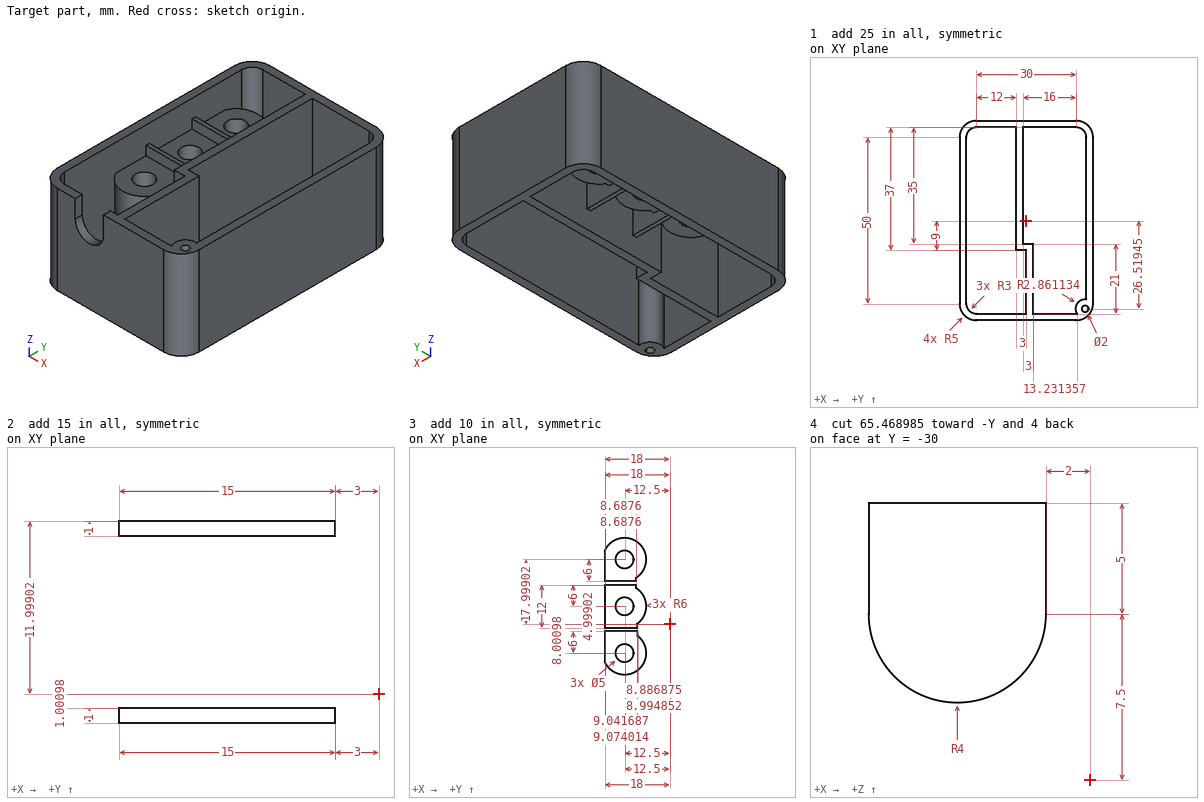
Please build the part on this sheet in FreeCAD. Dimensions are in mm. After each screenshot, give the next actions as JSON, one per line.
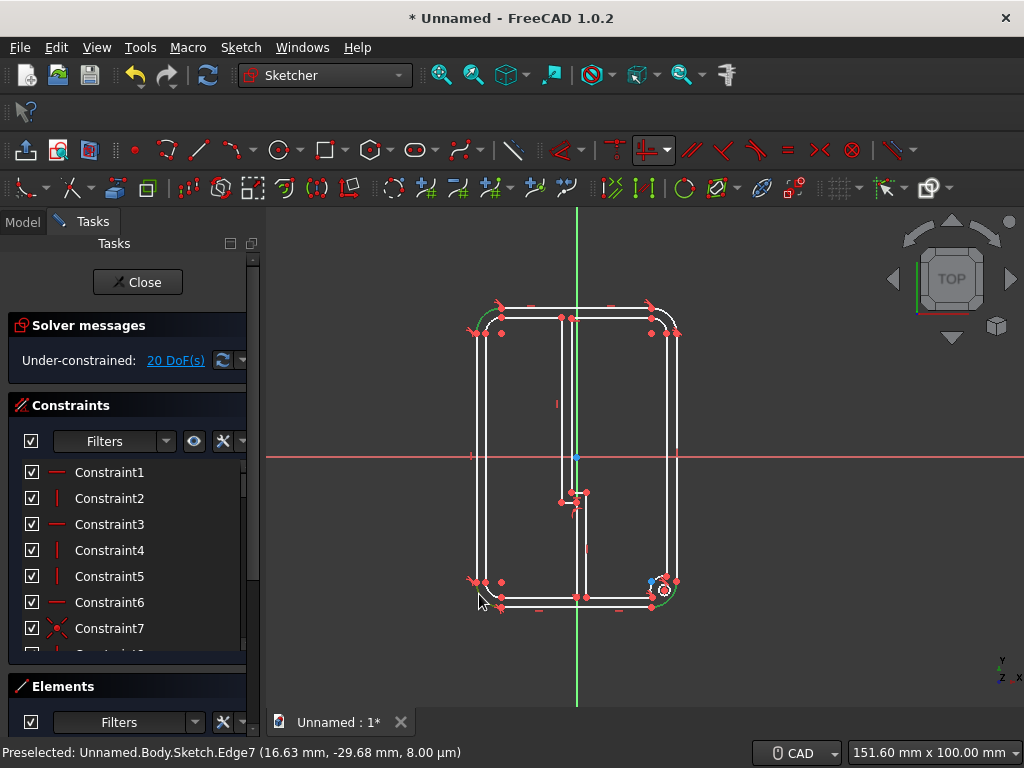
{"action": "scroll", "coordinate": [674, 322], "scroll_direction": "up", "scroll_amount": 2}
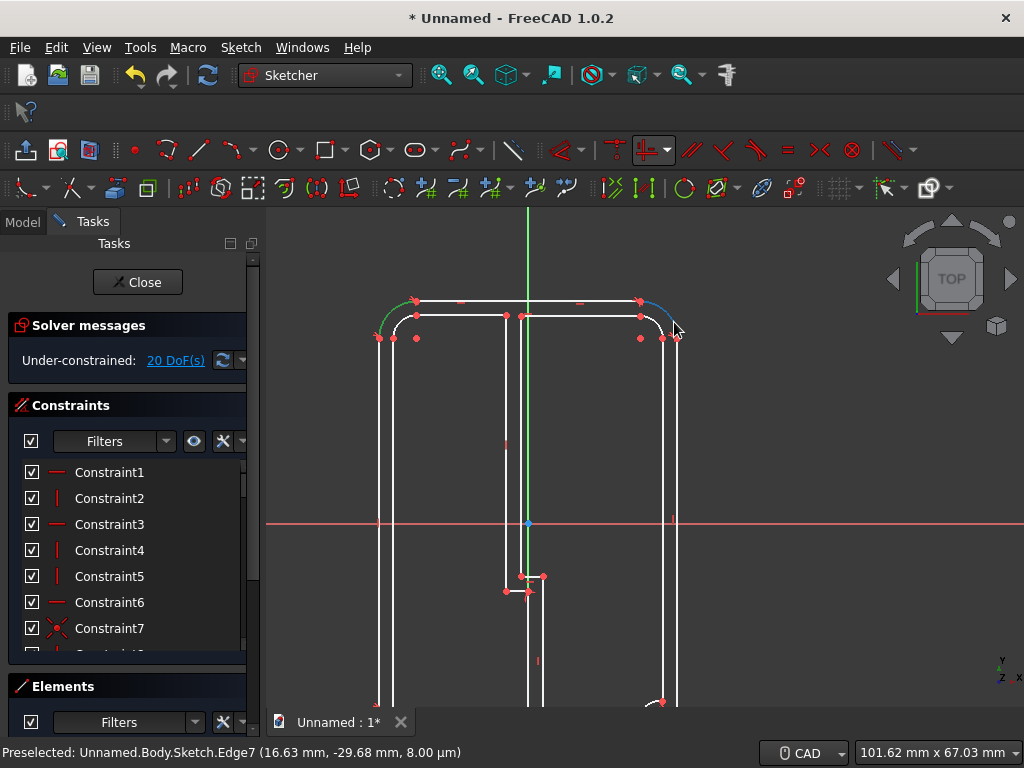
{"action": "left_click", "coordinate": [673, 322]}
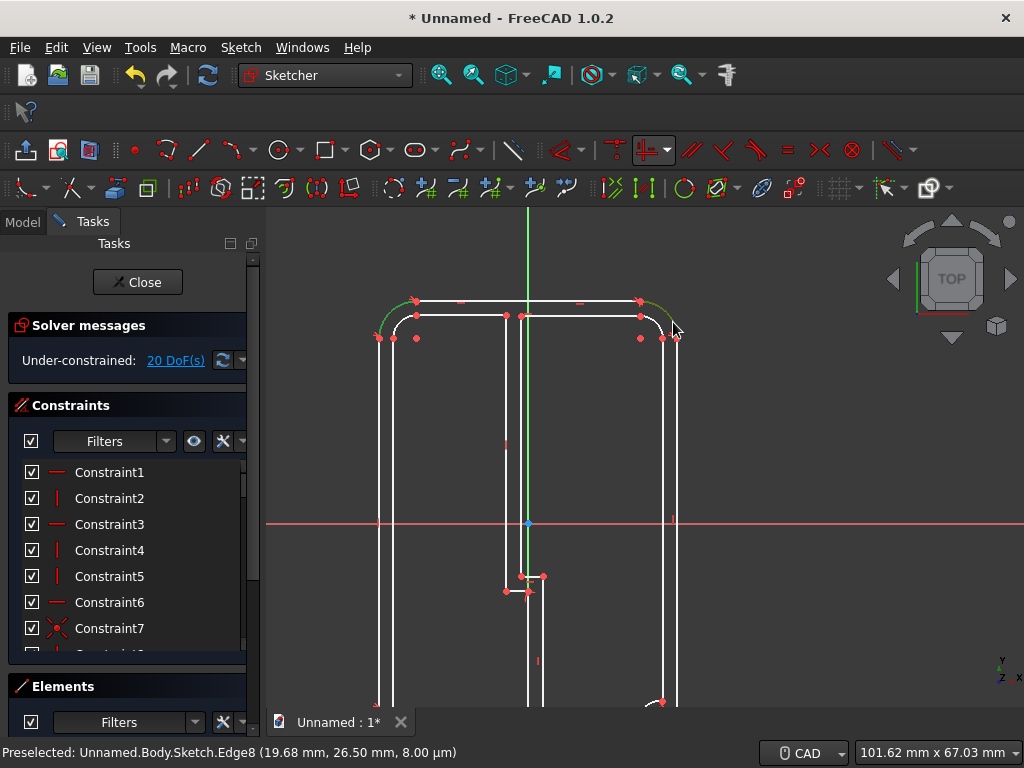
{"action": "left_click", "coordinate": [788, 150]}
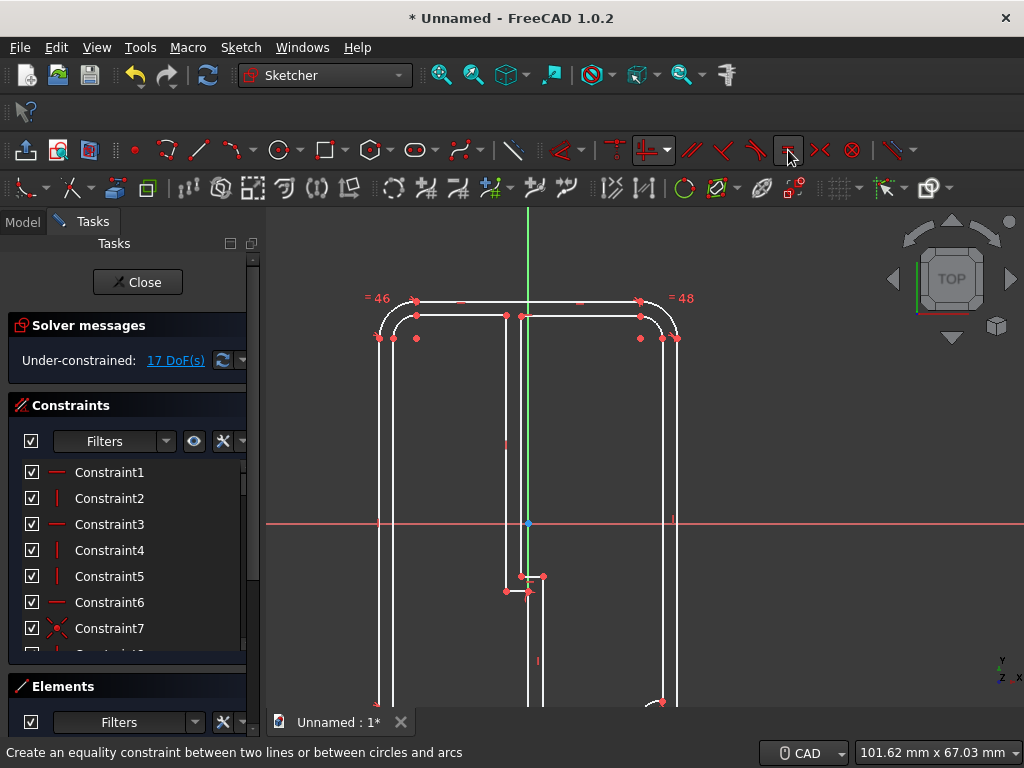
{"action": "scroll", "coordinate": [406, 318], "scroll_direction": "up", "scroll_amount": 2}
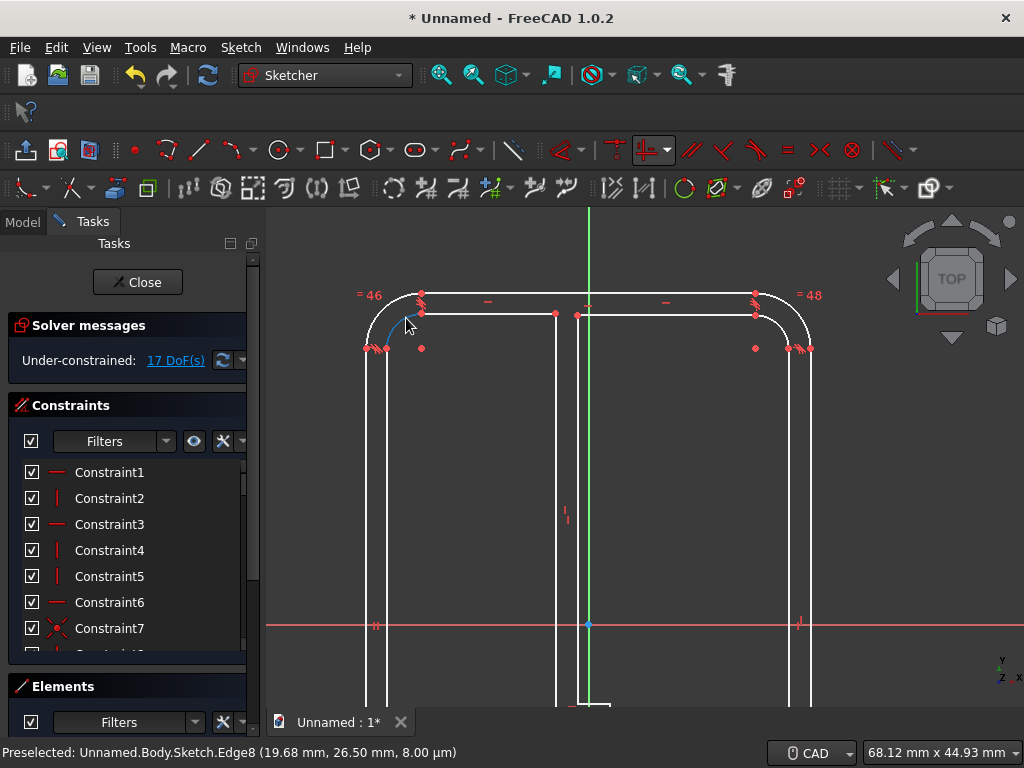
{"action": "left_click", "coordinate": [406, 318]}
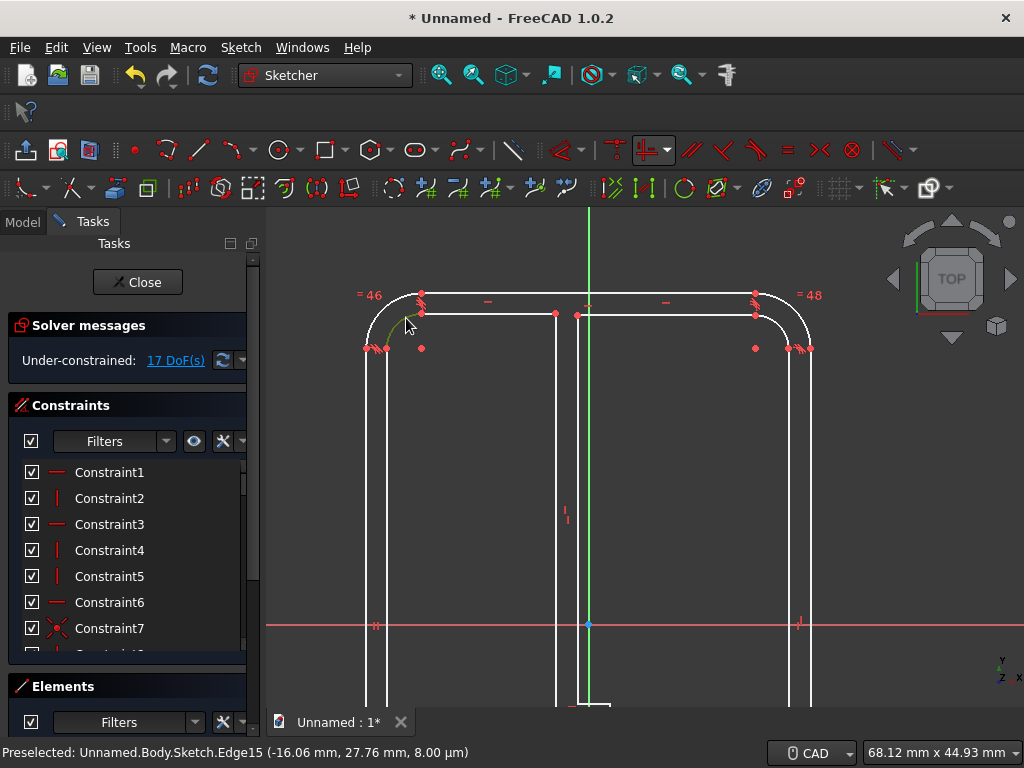
{"action": "left_click", "coordinate": [785, 334]}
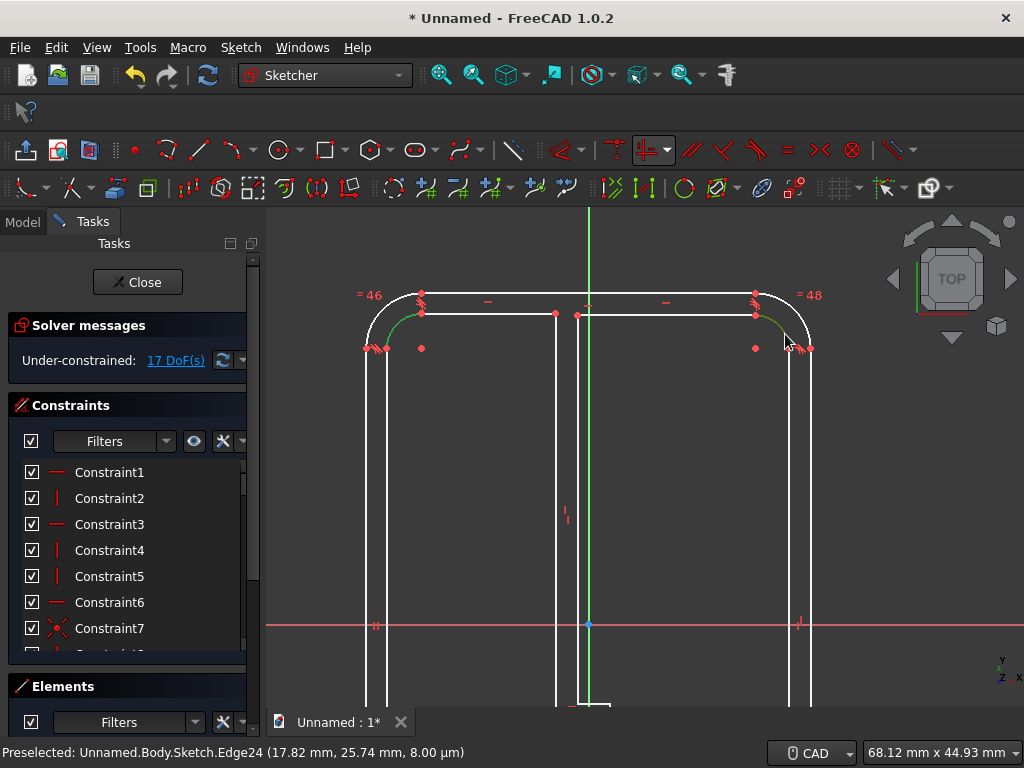
{"action": "left_click", "coordinate": [788, 150]}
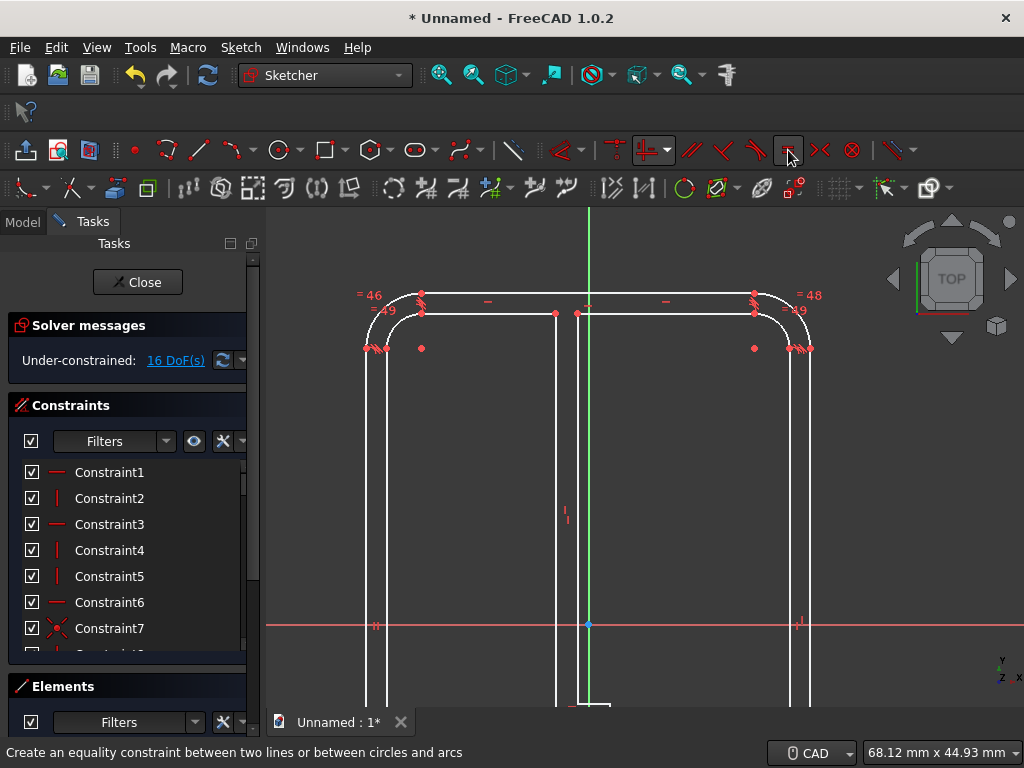
{"action": "left_click", "coordinate": [397, 299]}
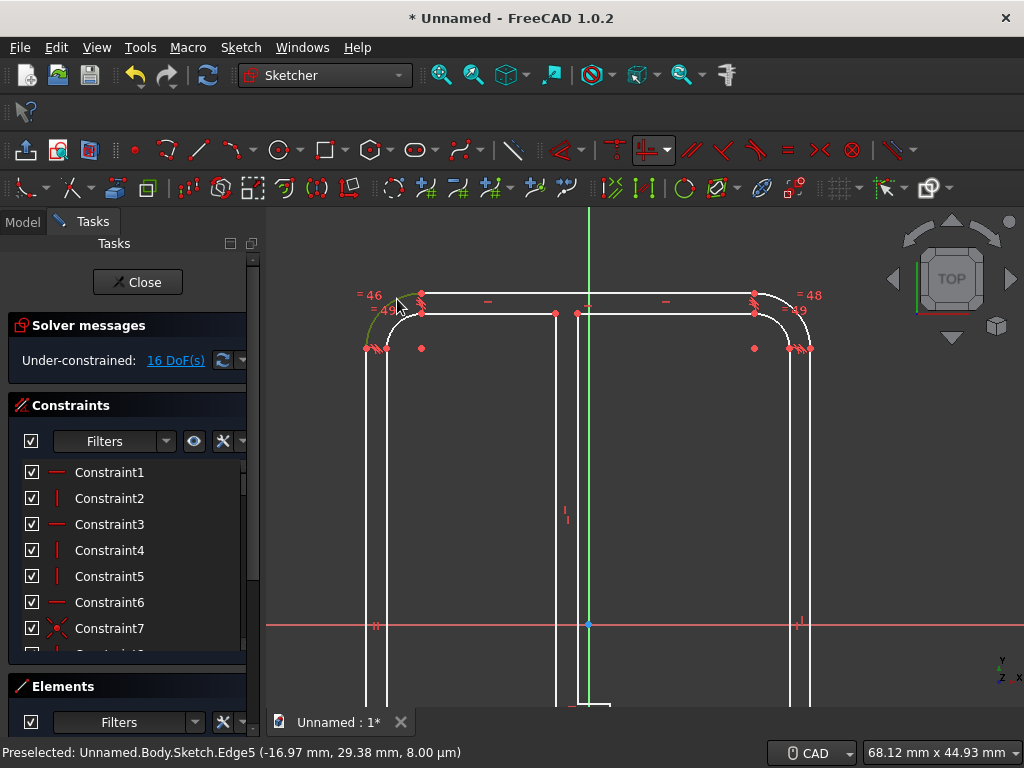
{"action": "left_click", "coordinate": [584, 150]}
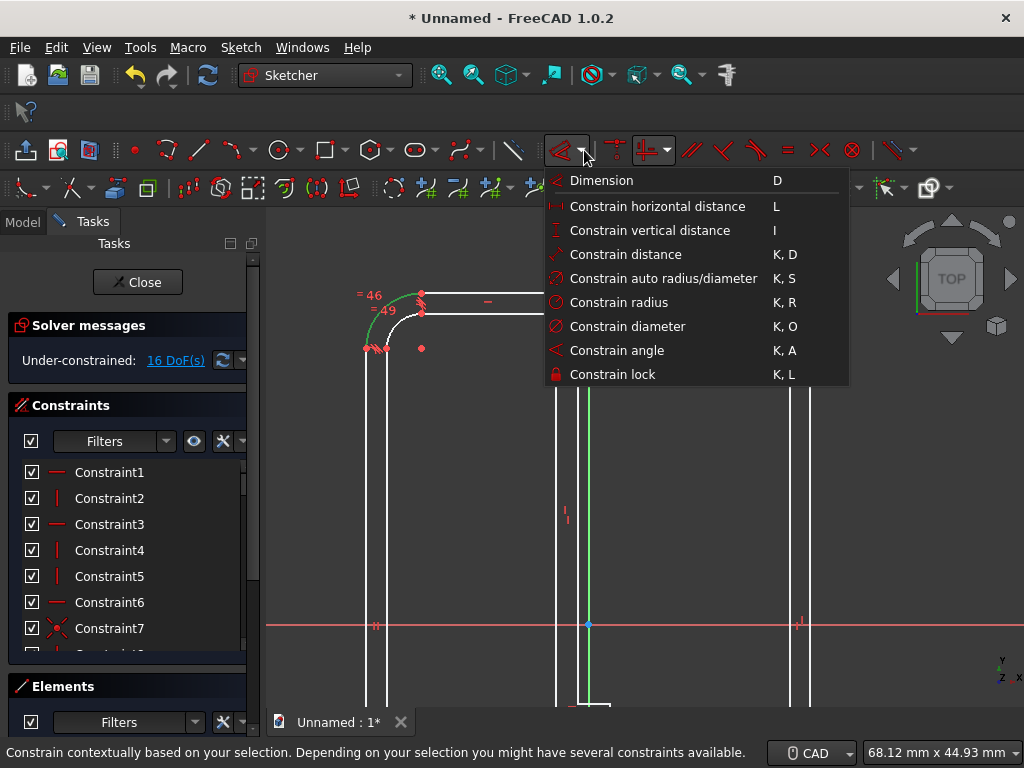
{"action": "left_click", "coordinate": [697, 302]}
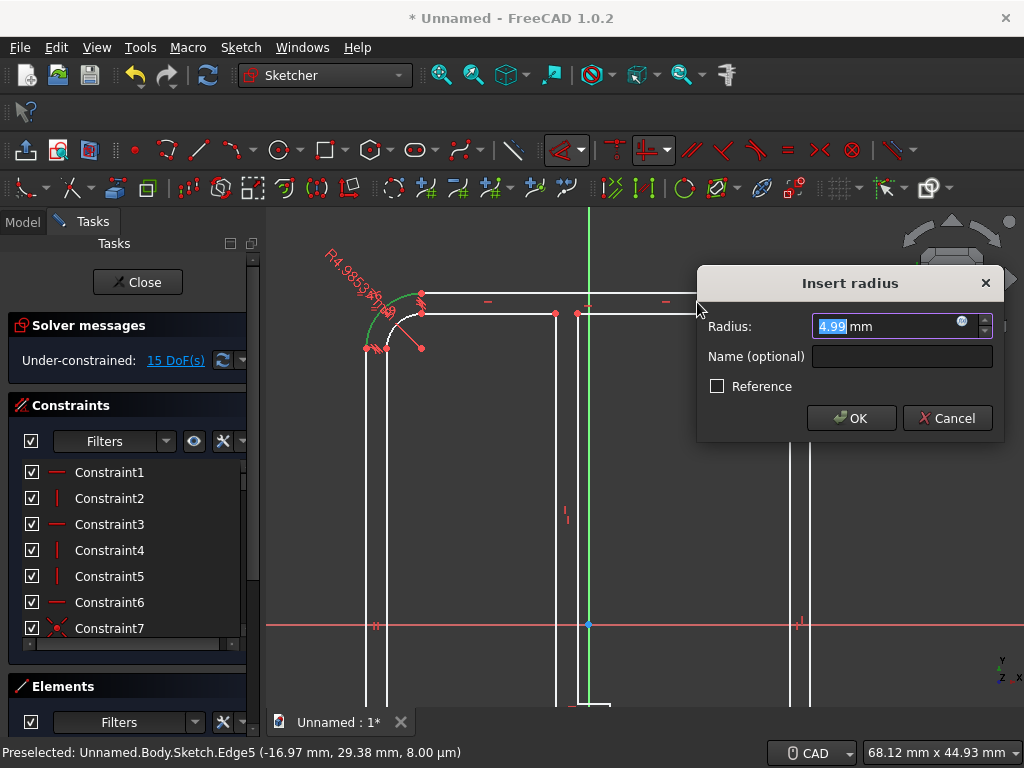
{"action": "type", "text": "5"}
{"action": "key", "text": "Return"}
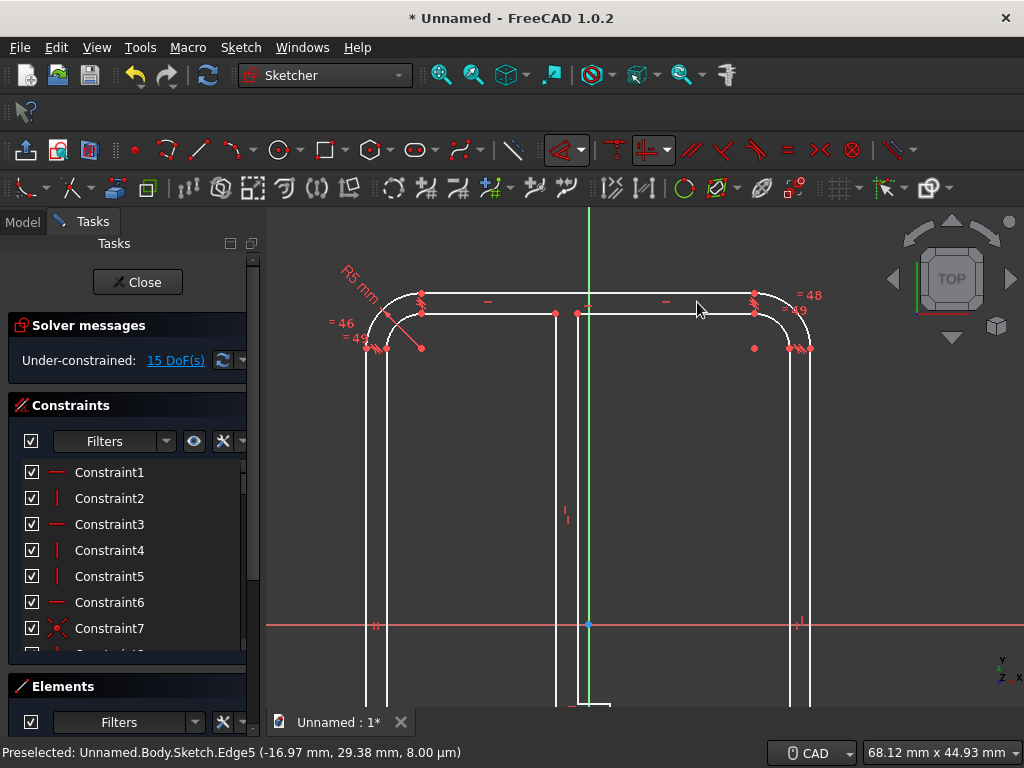
{"action": "left_click", "coordinate": [406, 318]}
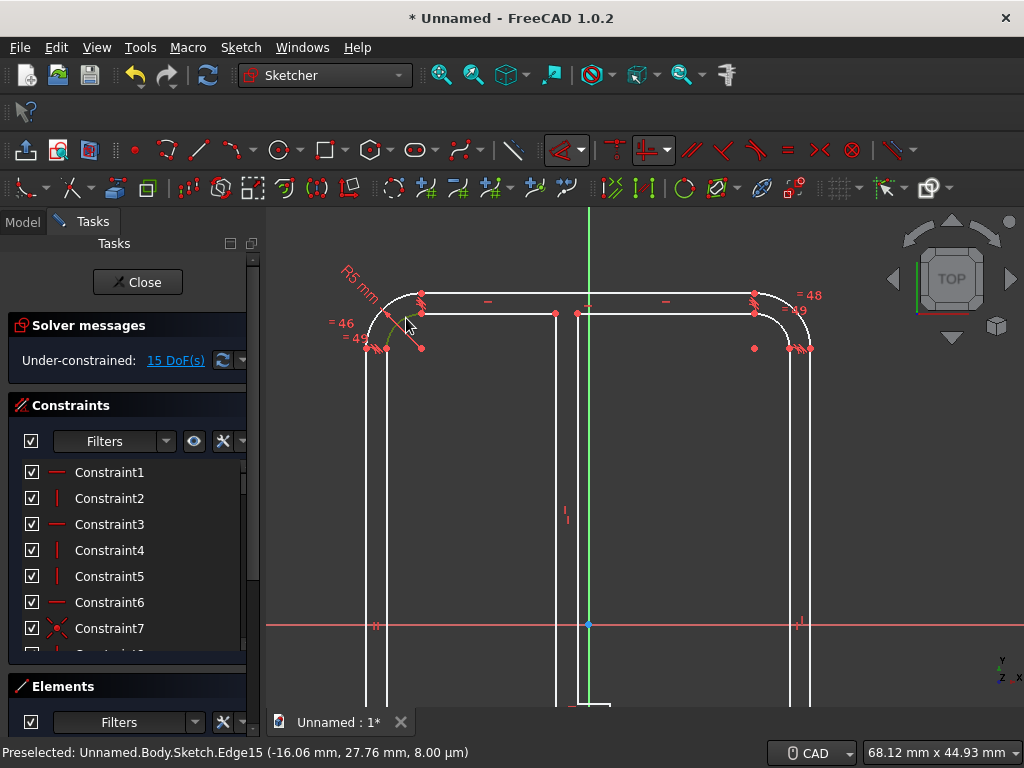
{"action": "key", "text": "k r"}